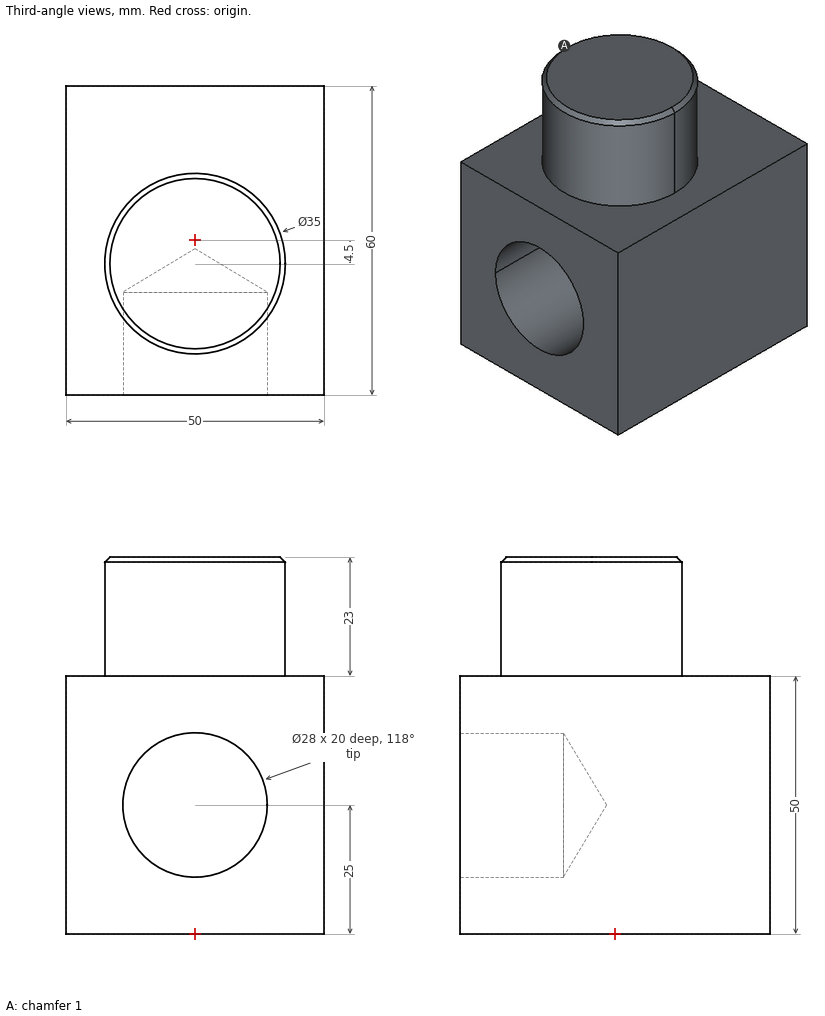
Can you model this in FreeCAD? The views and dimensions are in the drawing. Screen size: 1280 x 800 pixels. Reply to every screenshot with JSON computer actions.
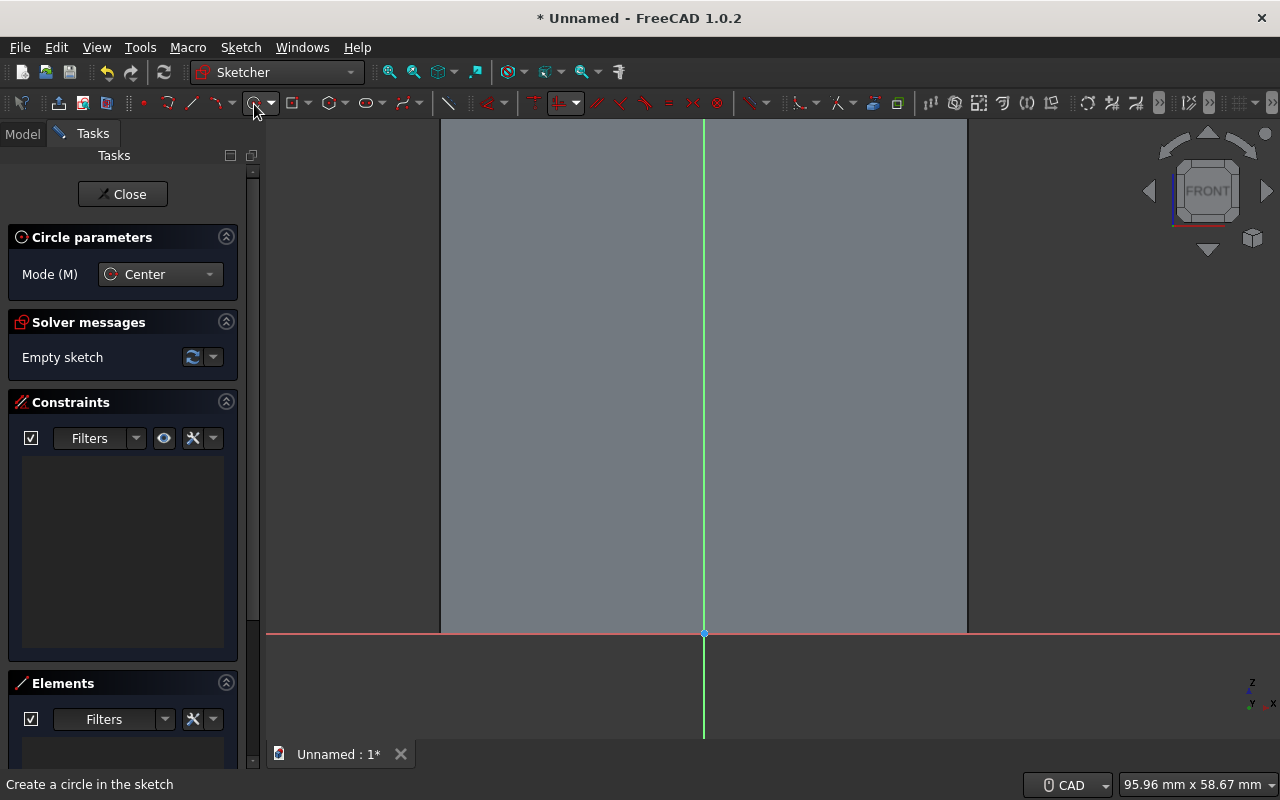
{"action": "left_click", "coordinate": [704, 370]}
{"action": "mouse_move", "coordinate": [809, 265]}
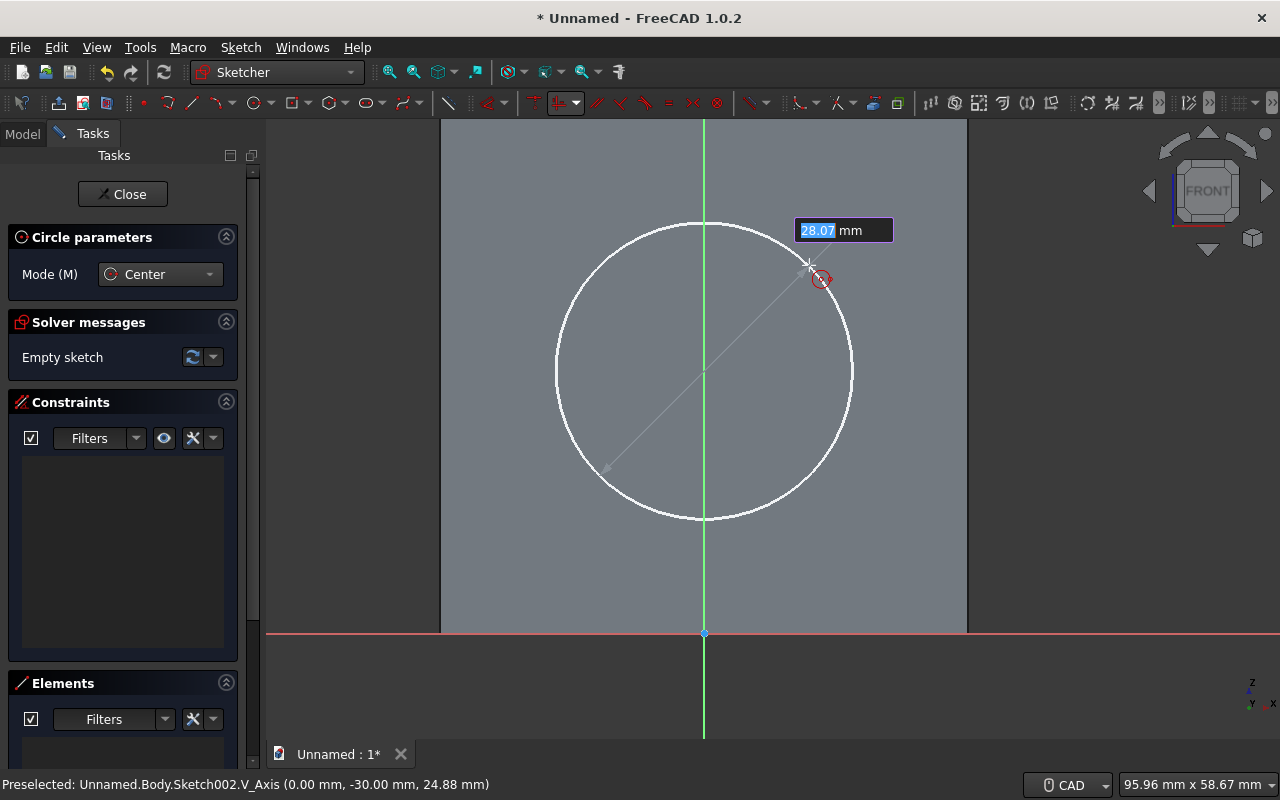
{"action": "type", "text": "28"}
{"action": "key", "text": "Return"}
{"action": "key", "text": "Escape"}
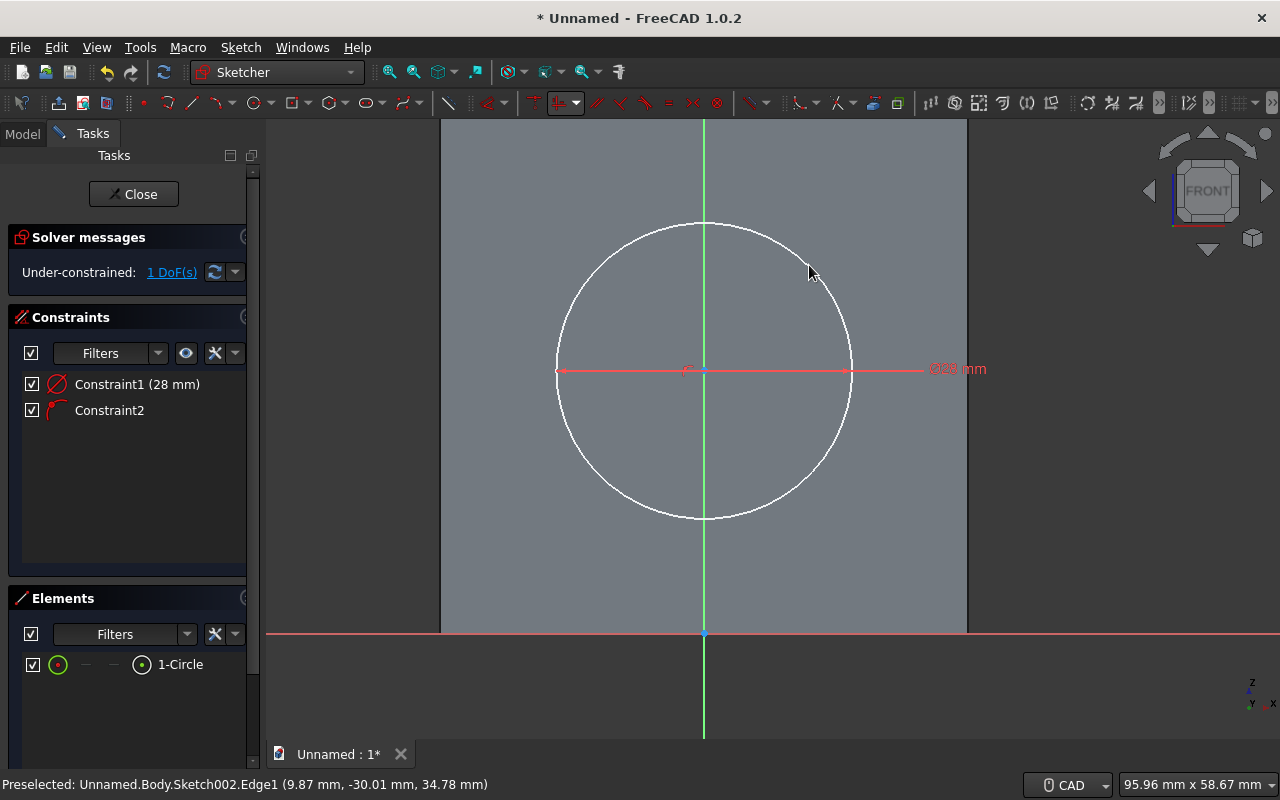
{"action": "left_click", "coordinate": [488, 104]}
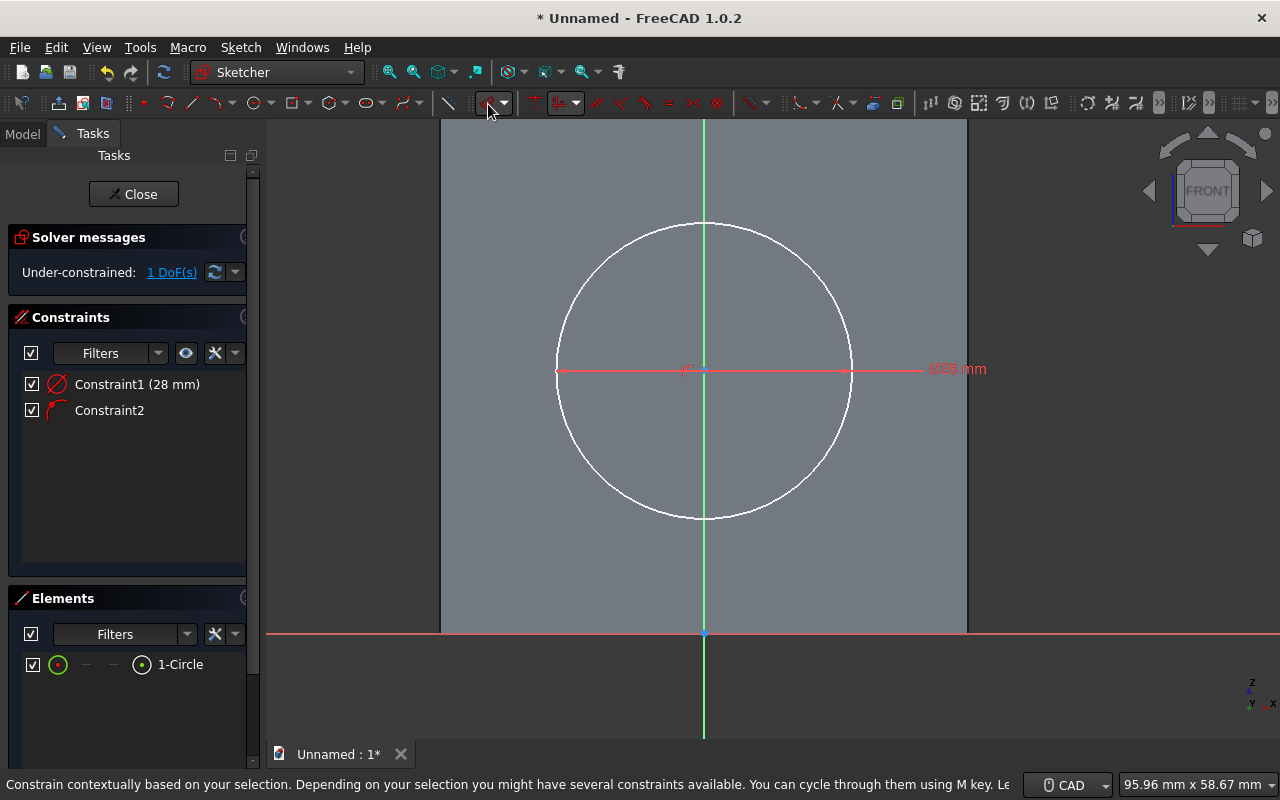
{"action": "left_click", "coordinate": [704, 371]}
{"action": "left_click", "coordinate": [738, 442]}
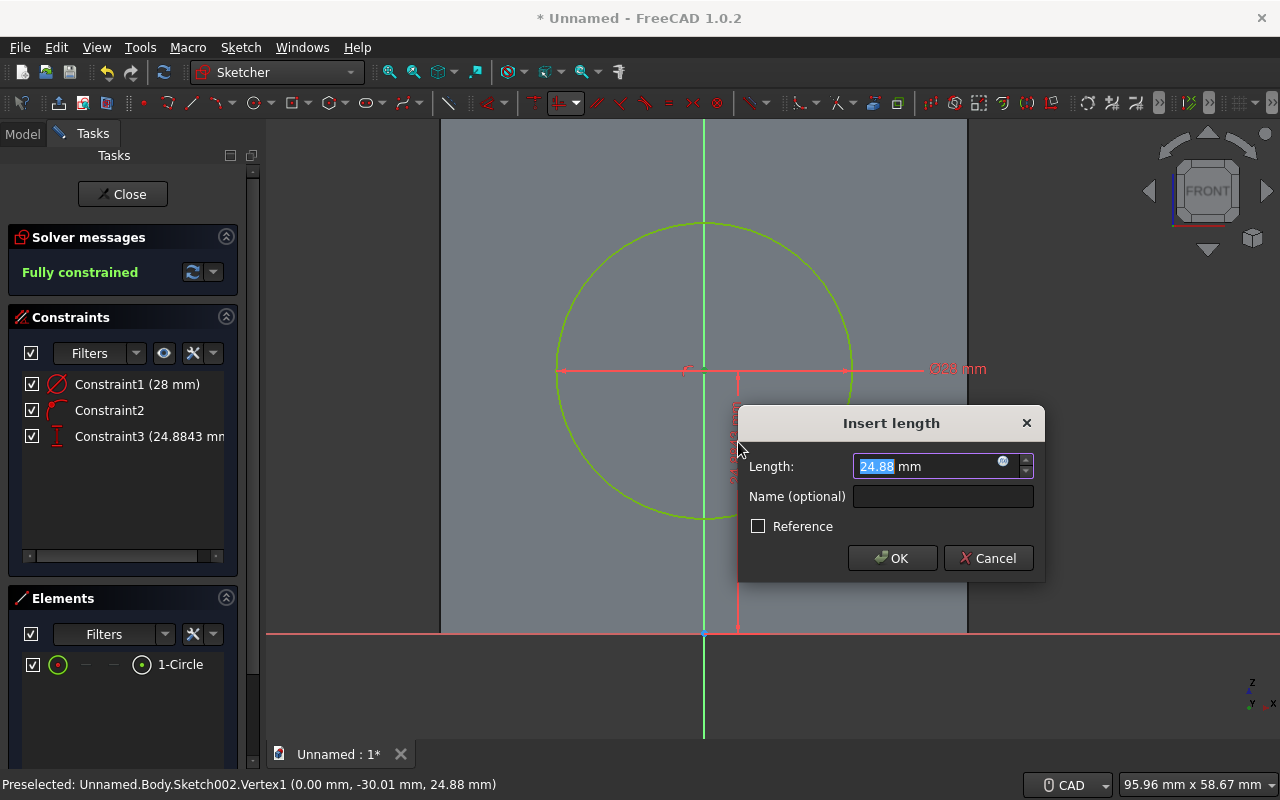
{"action": "type", "text": "25"}
{"action": "key", "text": "Return"}
{"action": "key", "text": "Escape"}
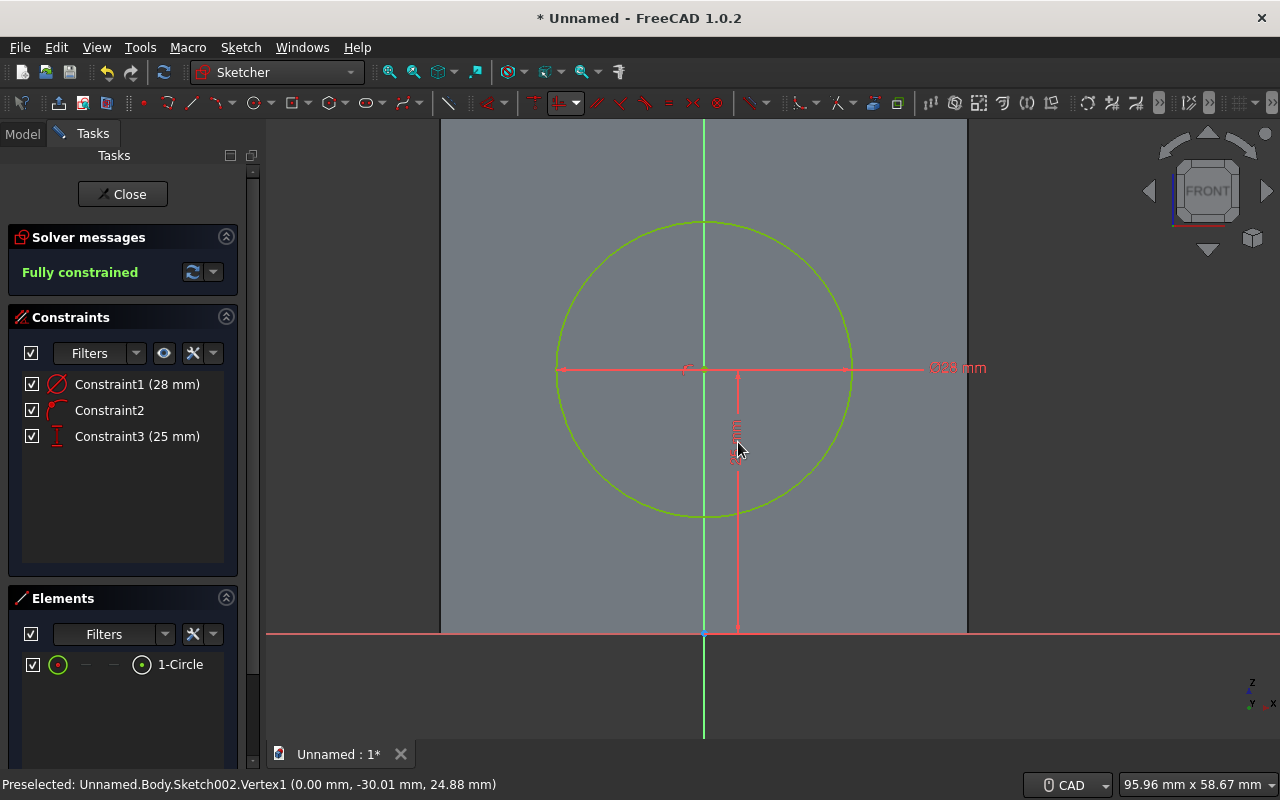
{"action": "left_click", "coordinate": [123, 194]}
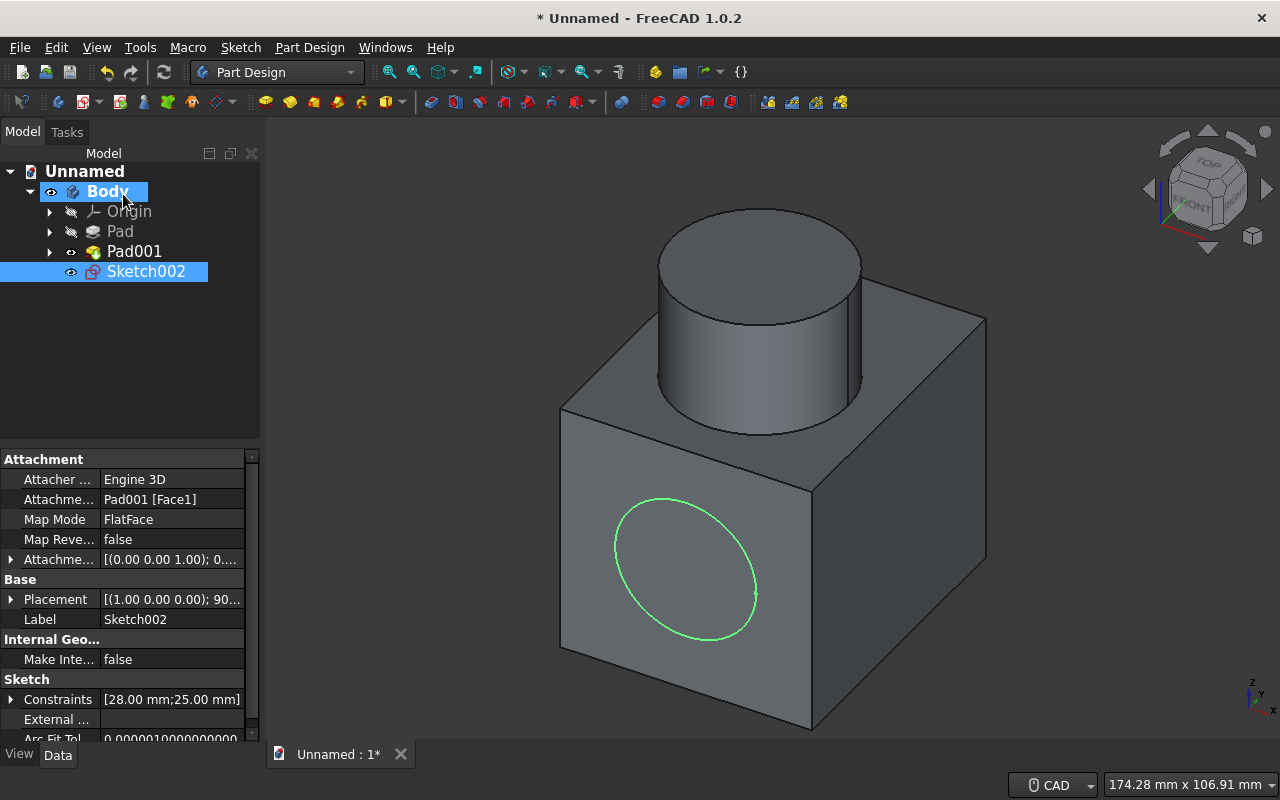
{"action": "left_click", "coordinate": [456, 102]}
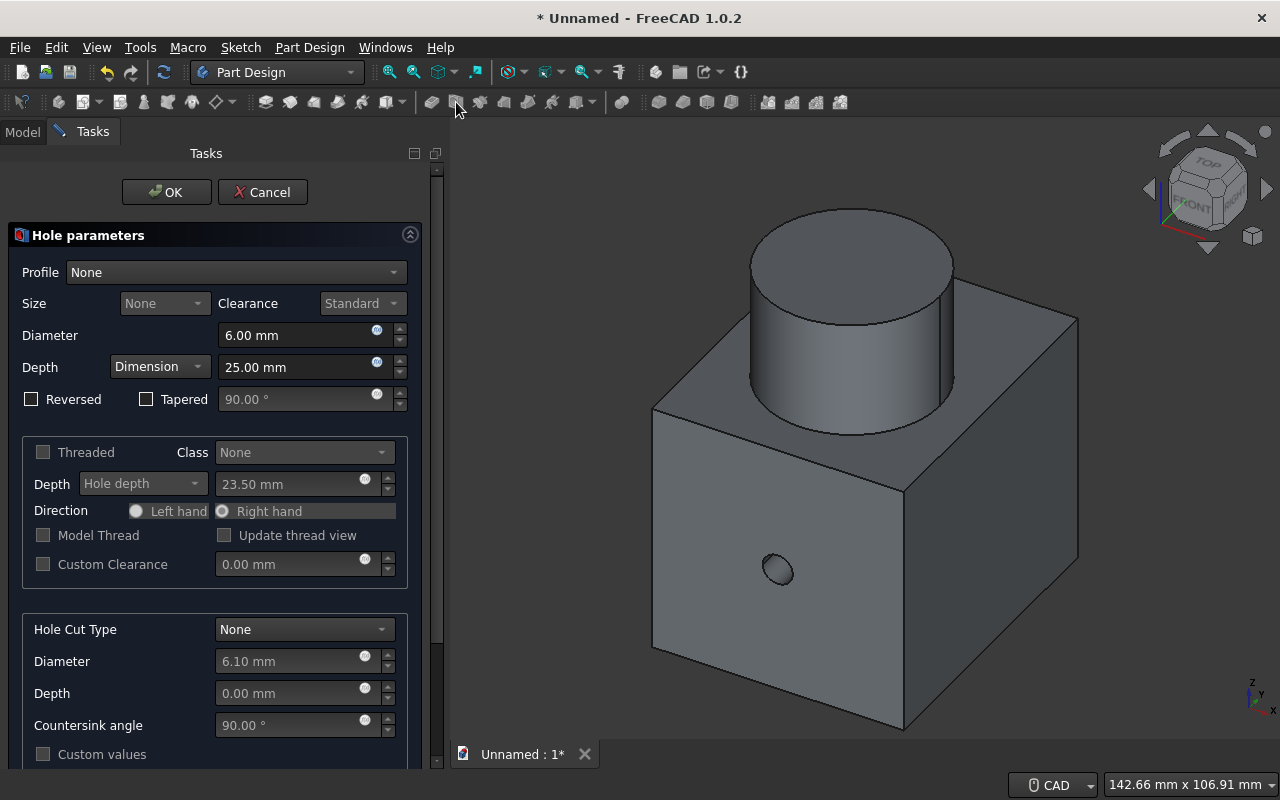
{"action": "triple_click", "coordinate": [305, 335]}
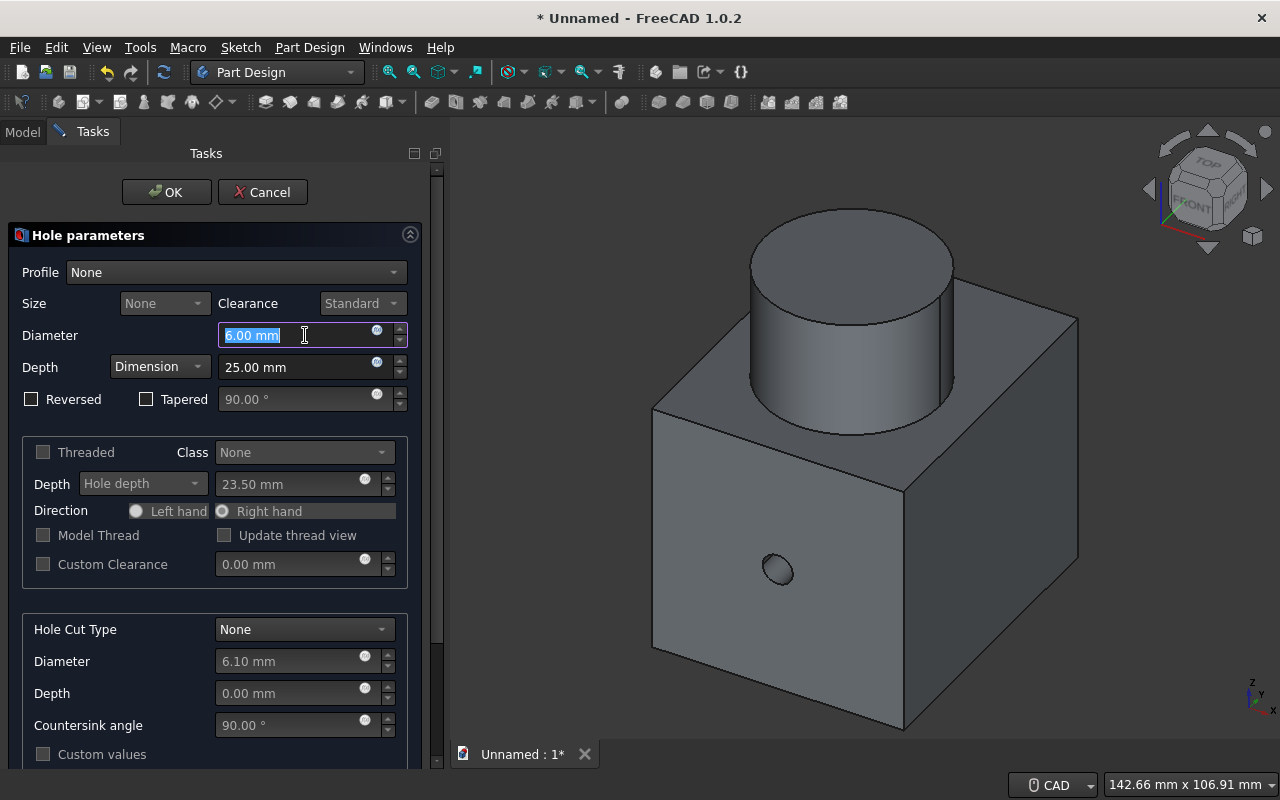
{"action": "type", "text": "28"}
{"action": "key", "text": "Tab"}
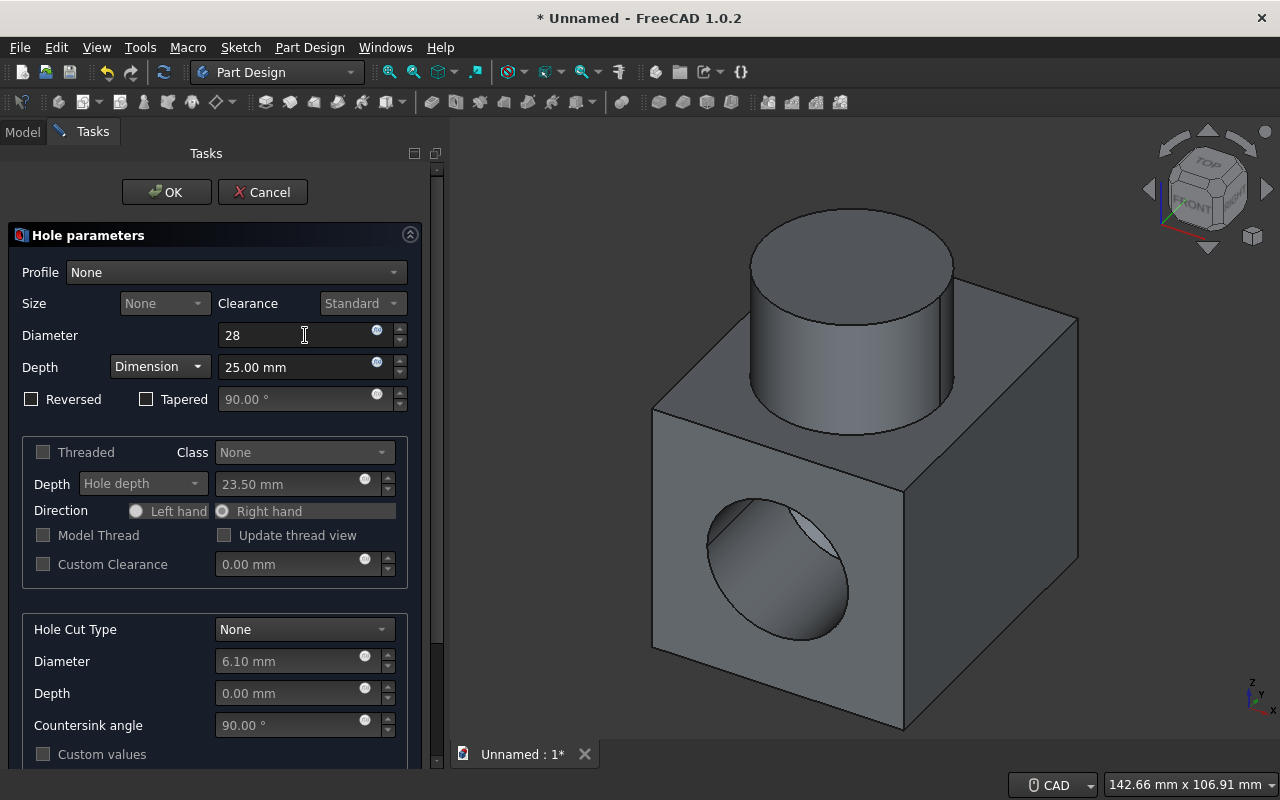
{"action": "triple_click", "coordinate": [305, 367]}